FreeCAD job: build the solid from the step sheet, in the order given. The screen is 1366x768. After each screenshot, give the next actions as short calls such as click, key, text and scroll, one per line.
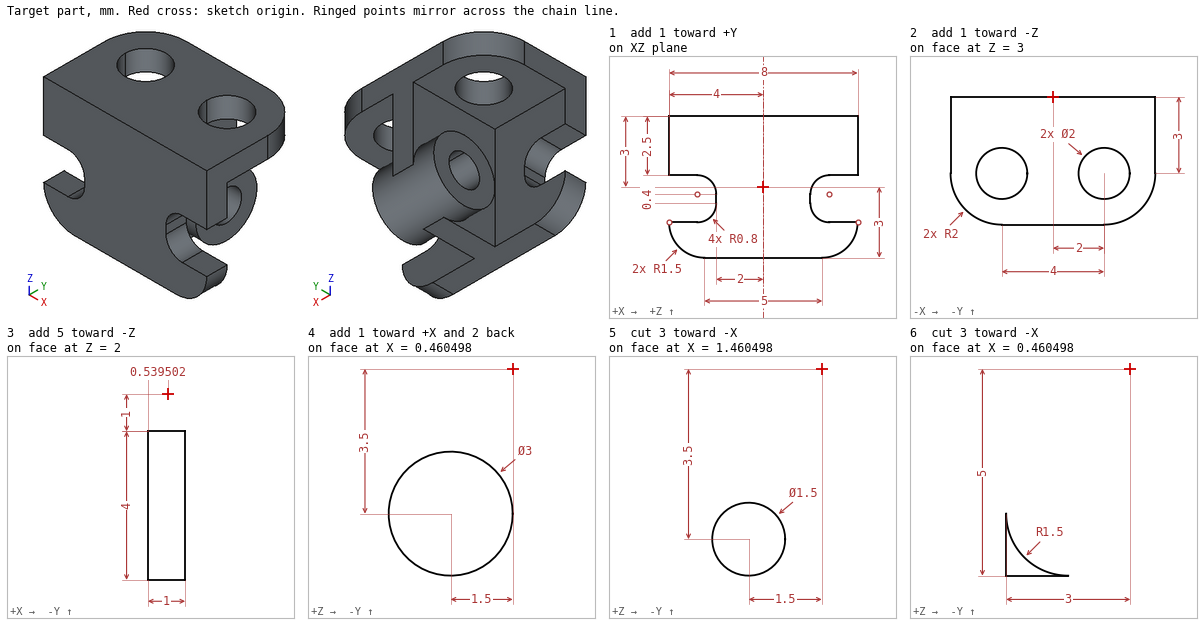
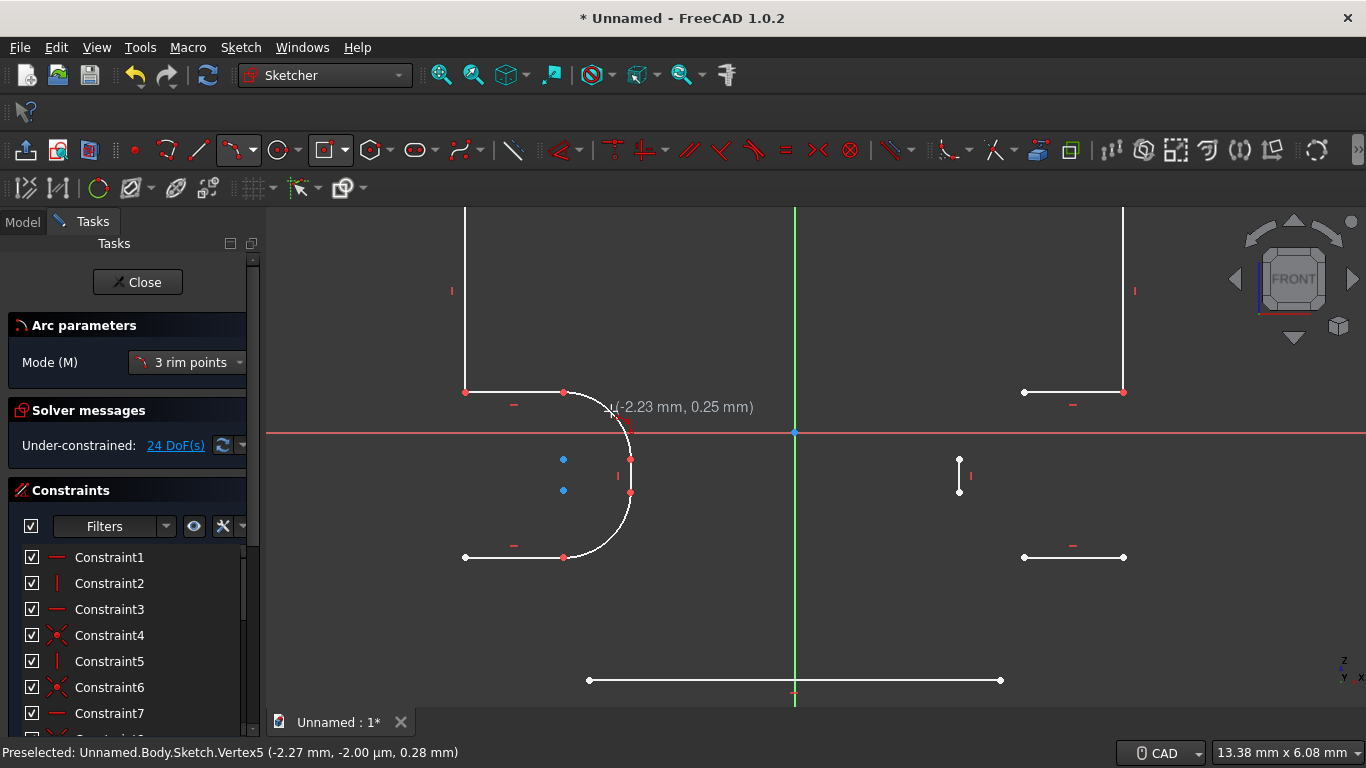
click(1025, 392)
click(959, 459)
click(978, 411)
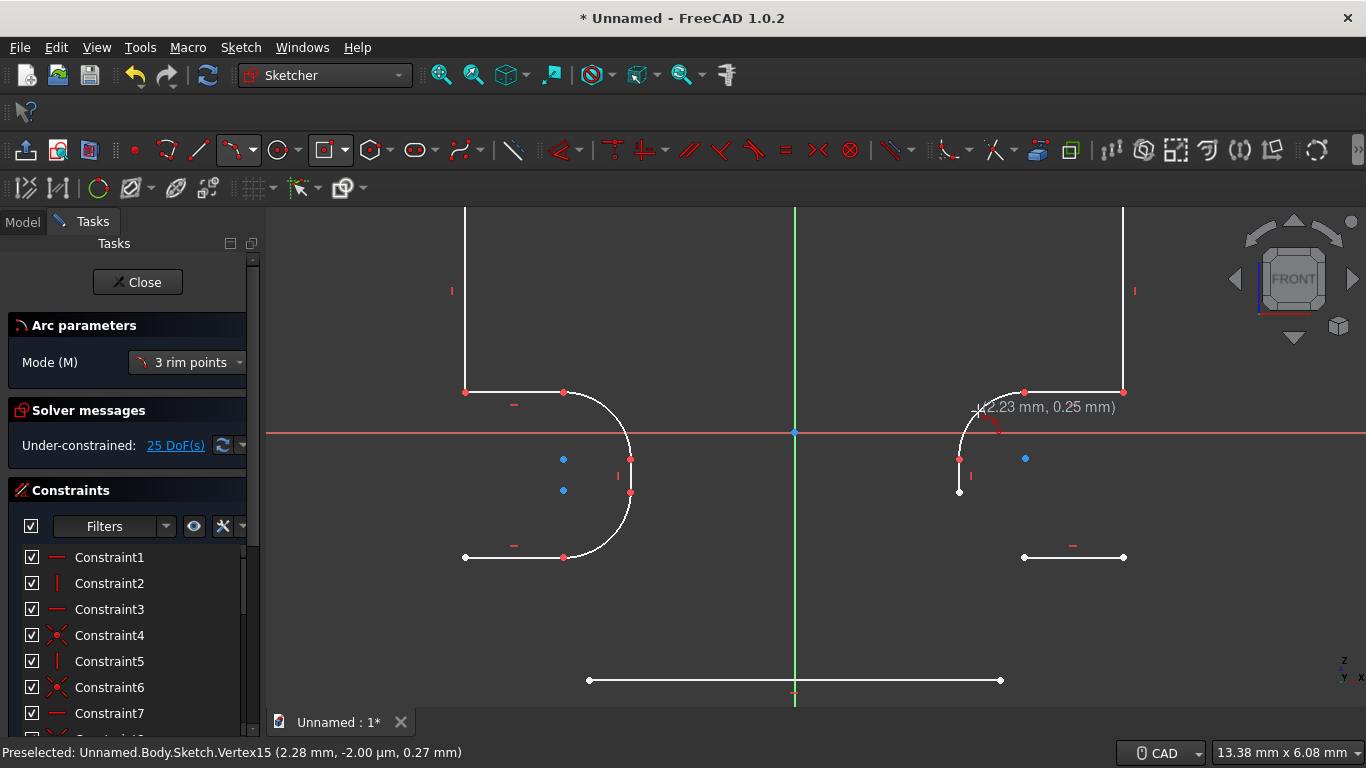
click(959, 492)
click(1025, 558)
click(978, 537)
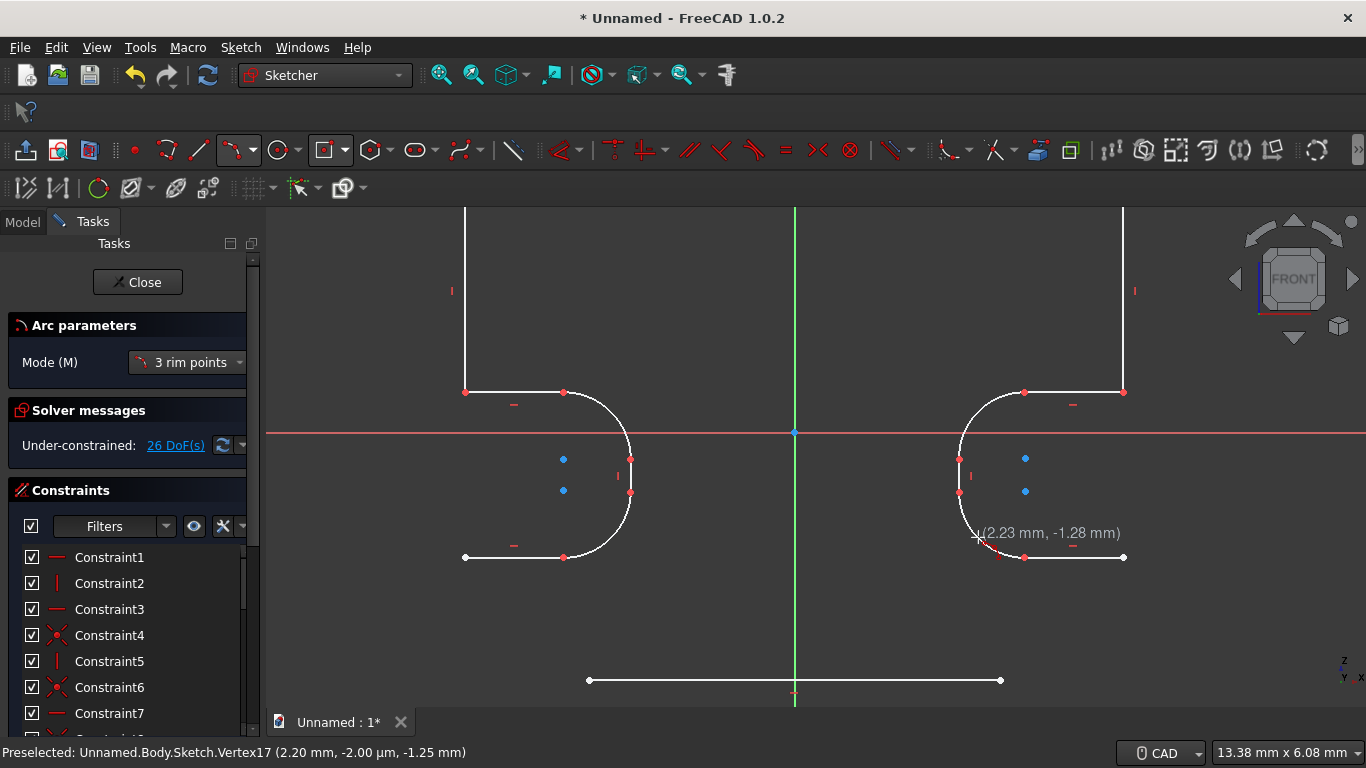
click(1123, 558)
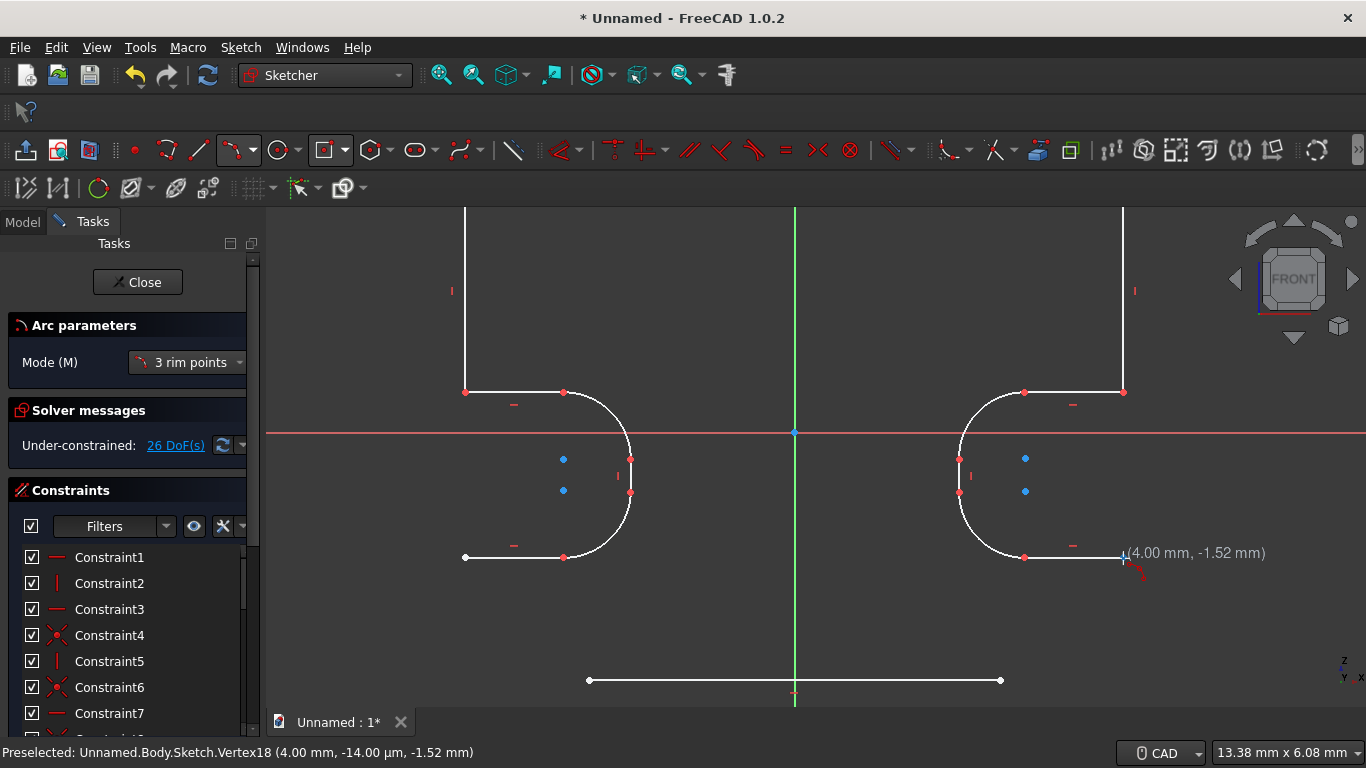
scroll(652, 507, down, 2)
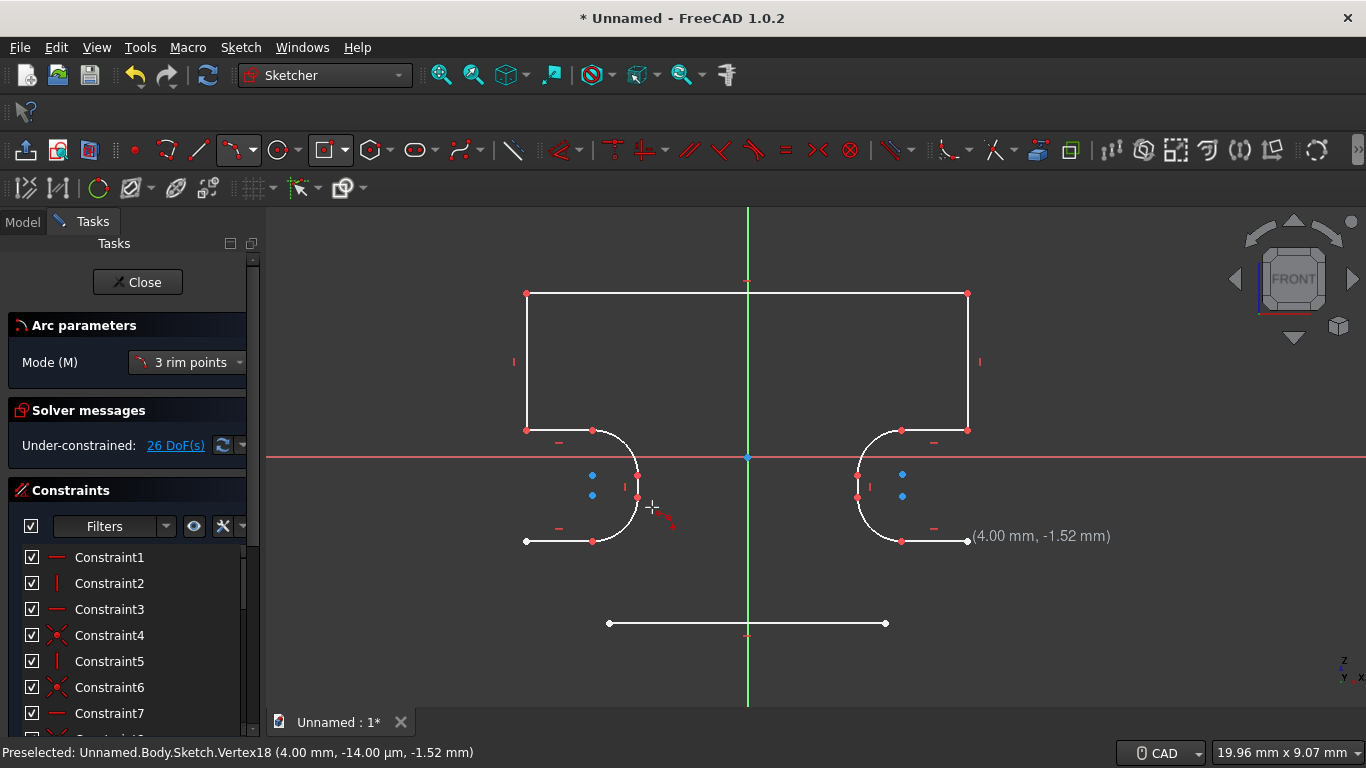
click(886, 623)
click(944, 598)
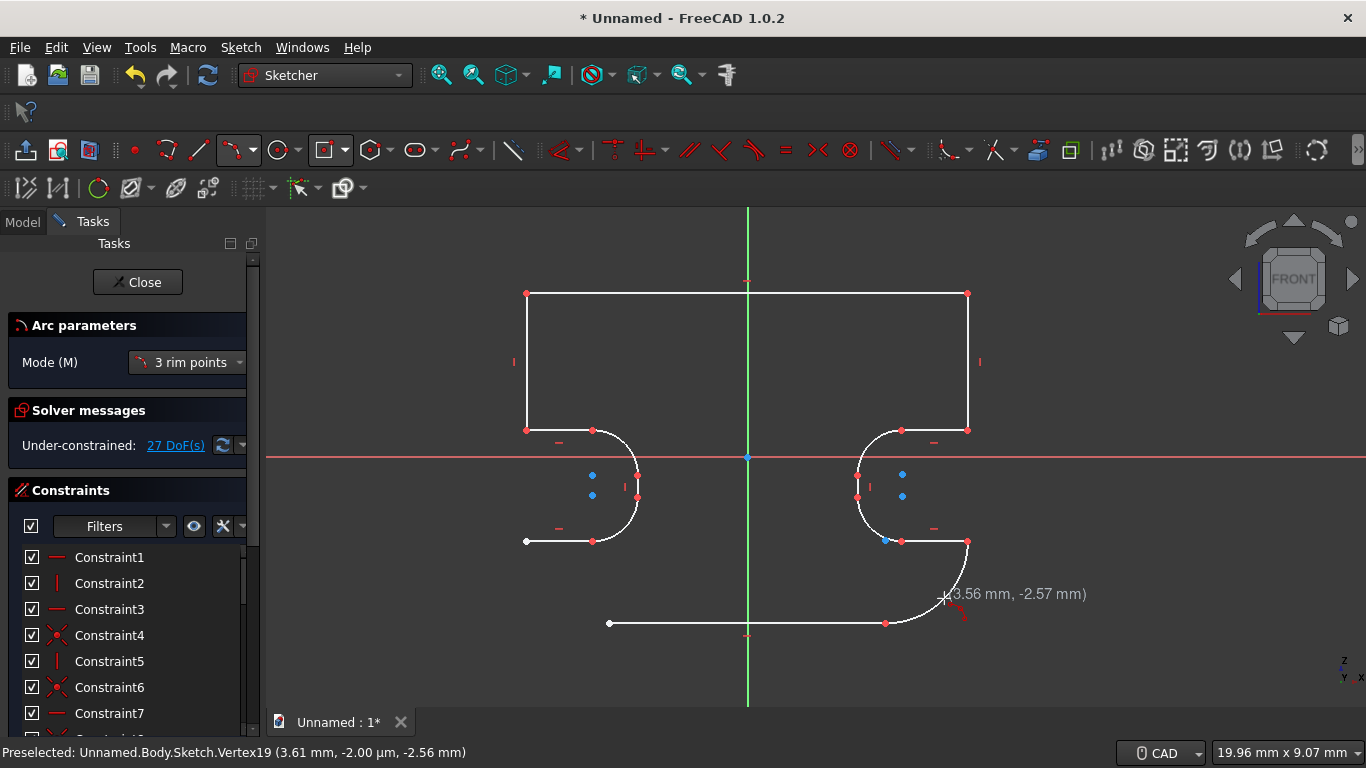
click(610, 623)
click(527, 541)
click(551, 598)
key(Escape)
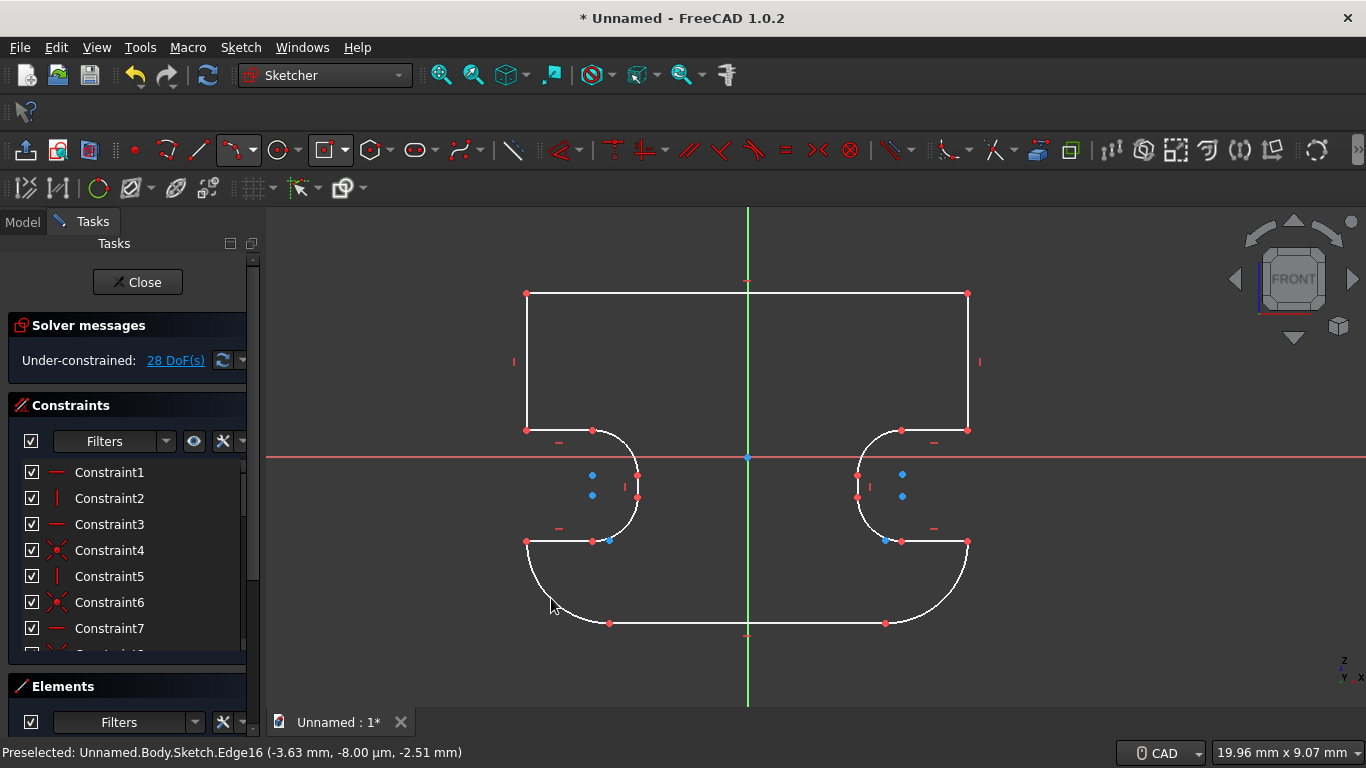
click(547, 541)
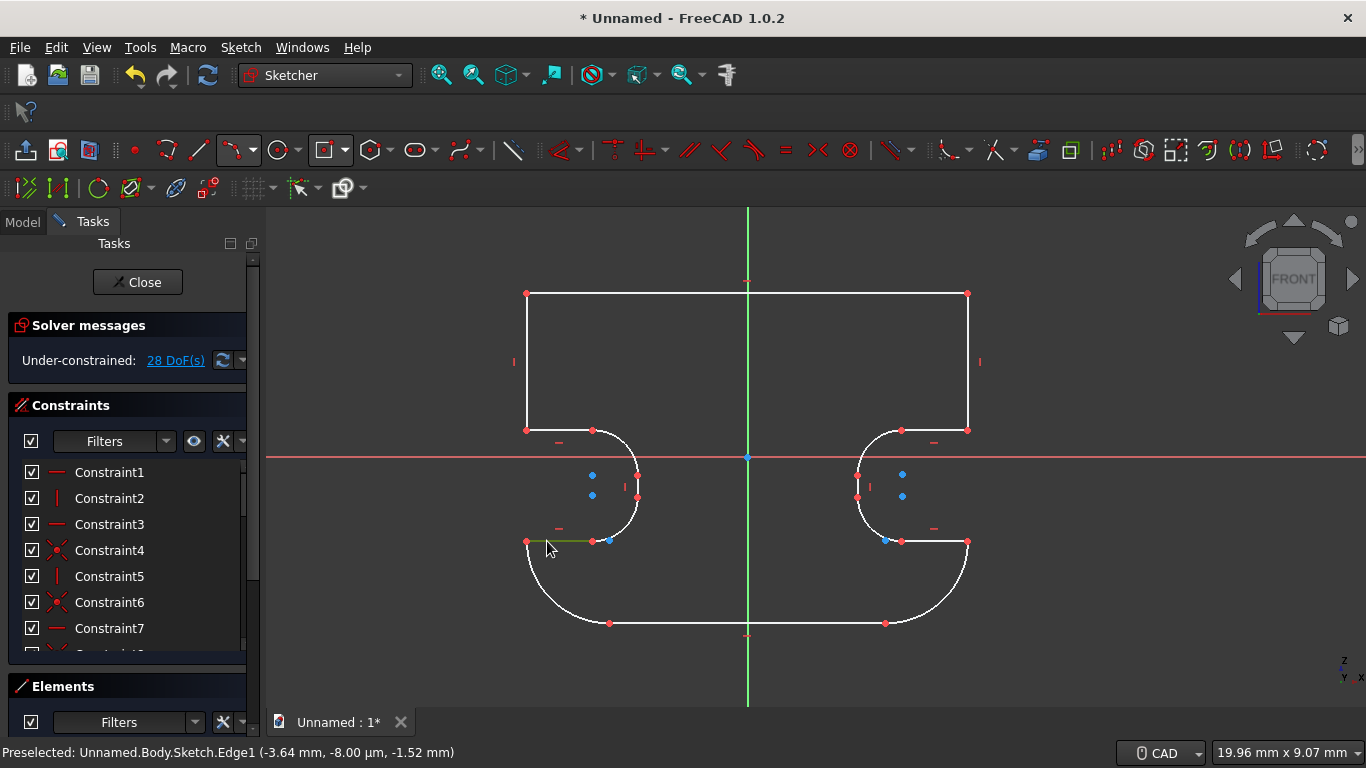
click(613, 536)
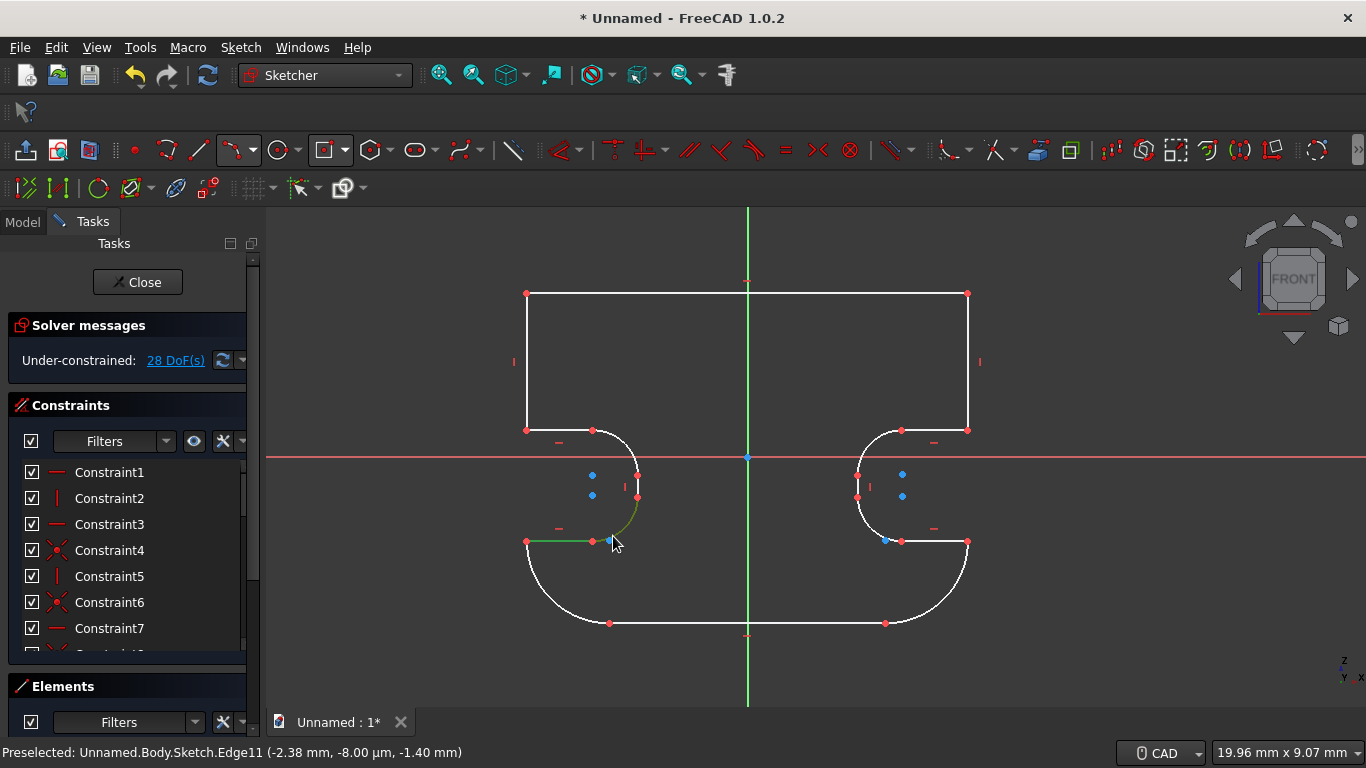
click(754, 150)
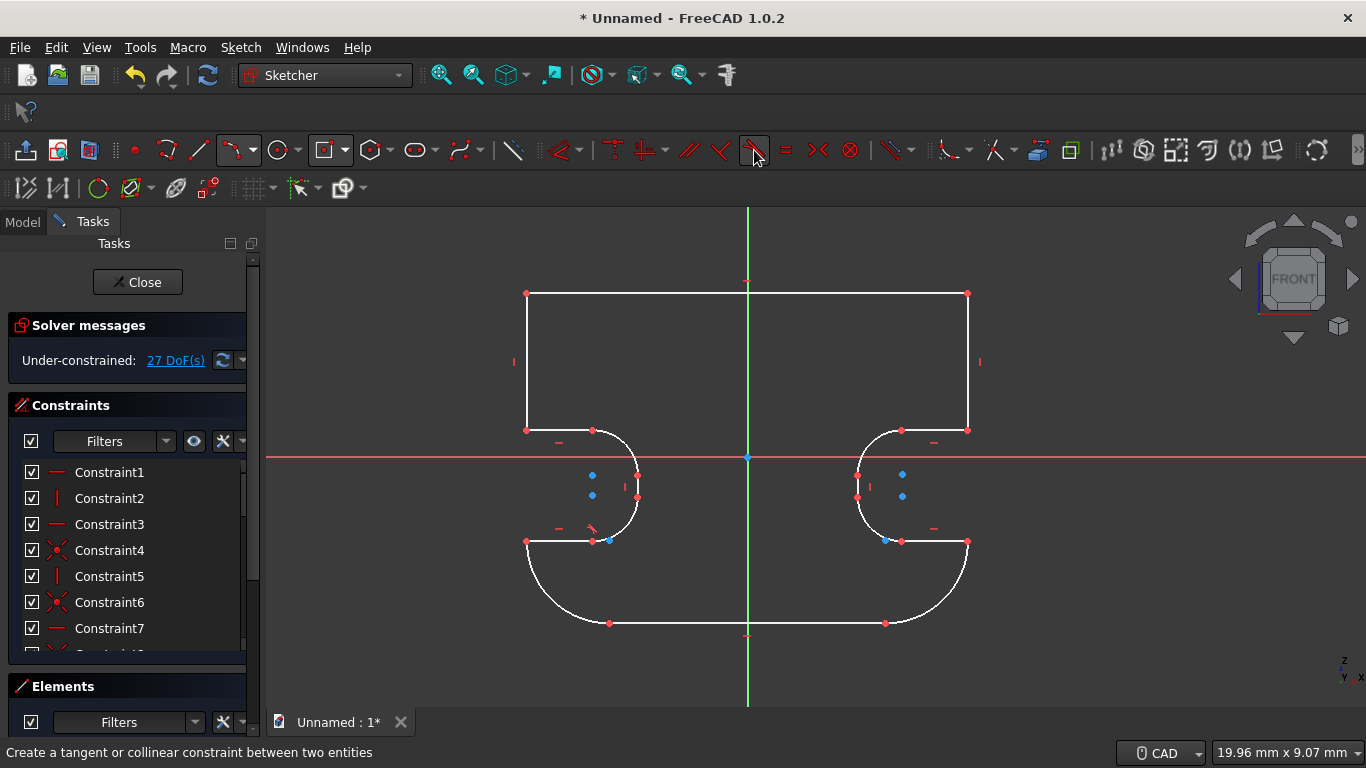
scroll(638, 486, up, 2)